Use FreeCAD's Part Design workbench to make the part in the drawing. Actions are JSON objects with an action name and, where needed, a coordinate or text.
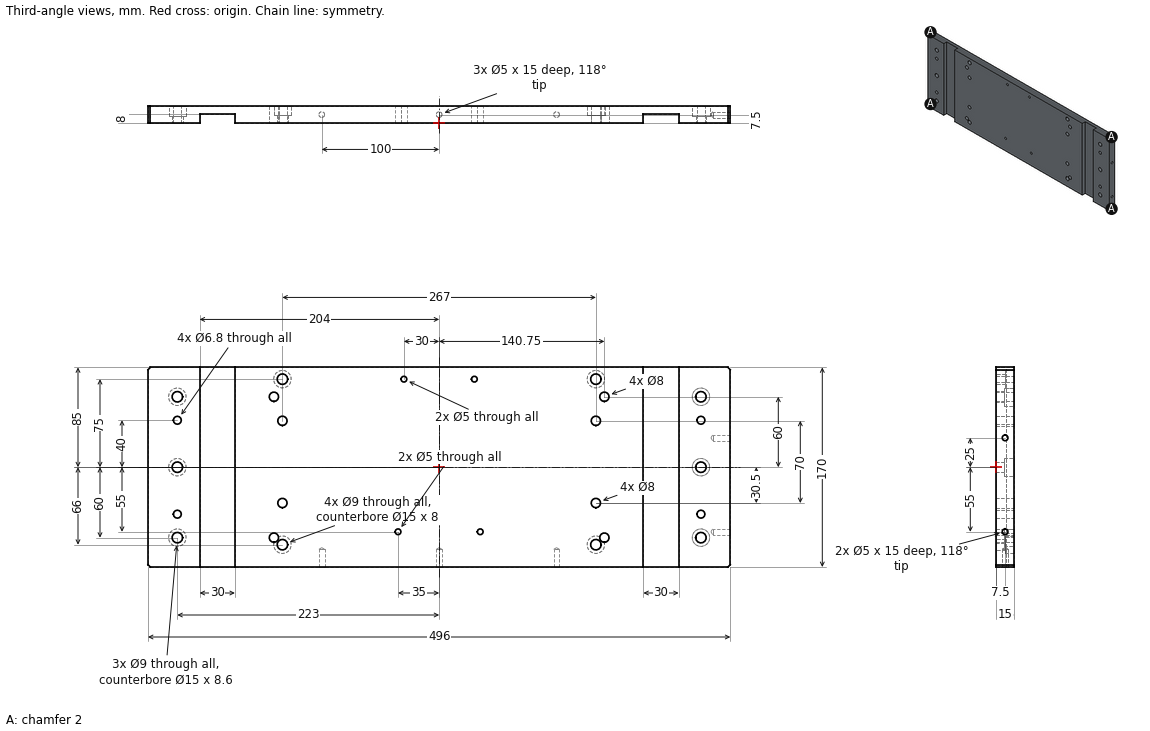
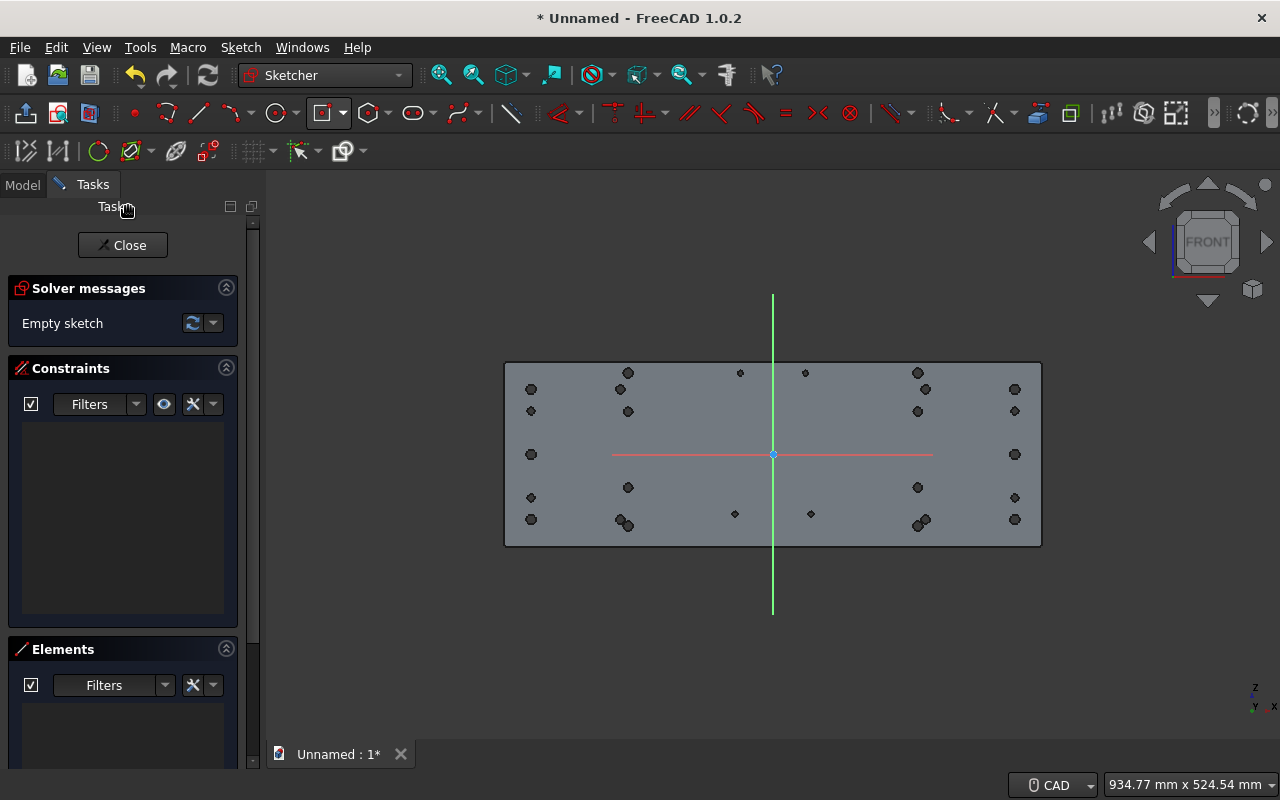
{"action": "left_click", "coordinate": [346, 114]}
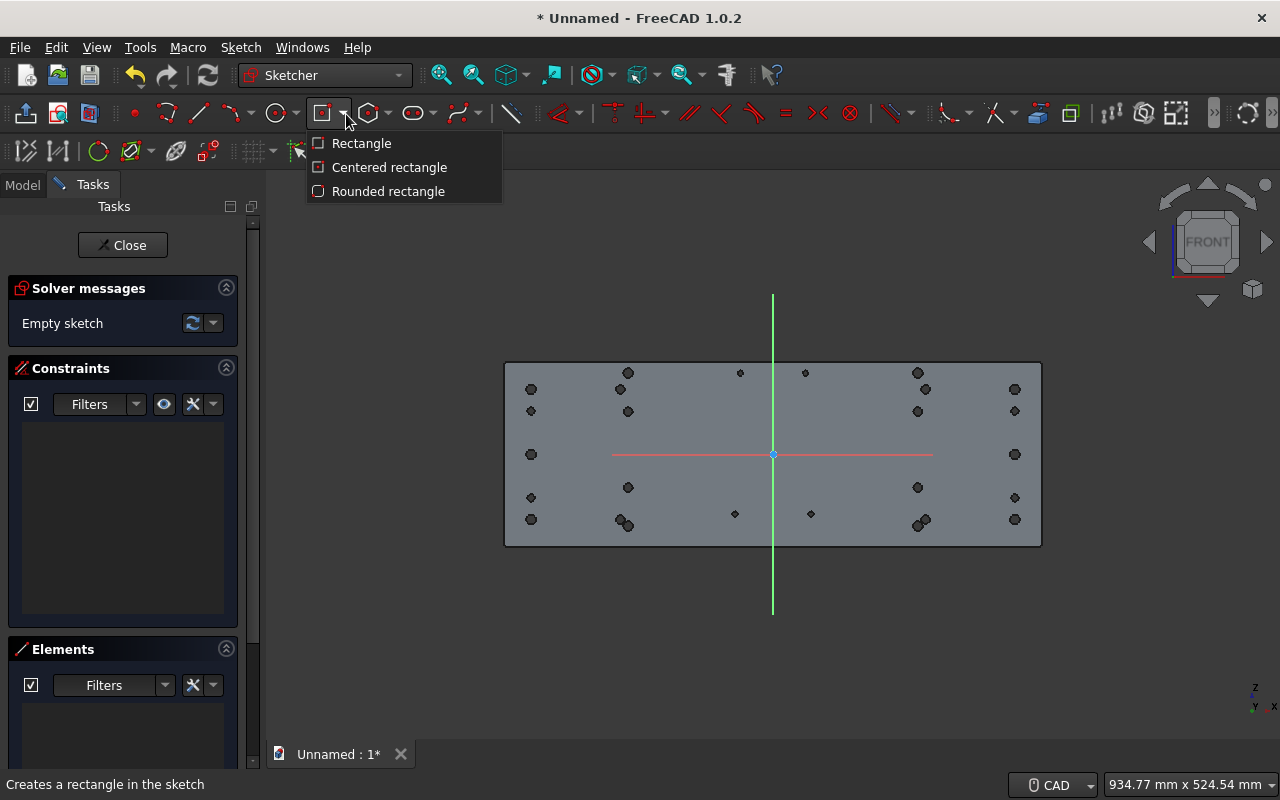
{"action": "left_click", "coordinate": [404, 143]}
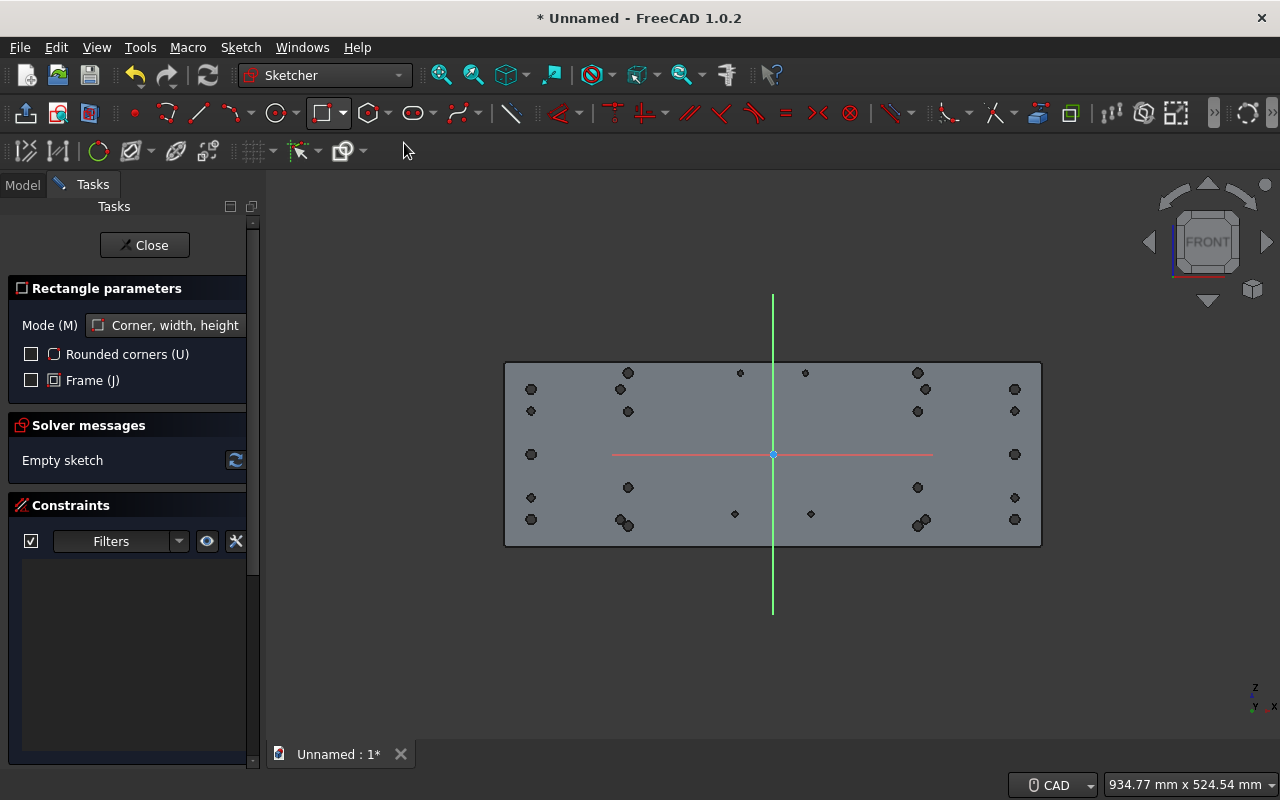
{"action": "left_click", "coordinate": [552, 362]}
{"action": "mouse_move", "coordinate": [584, 547]}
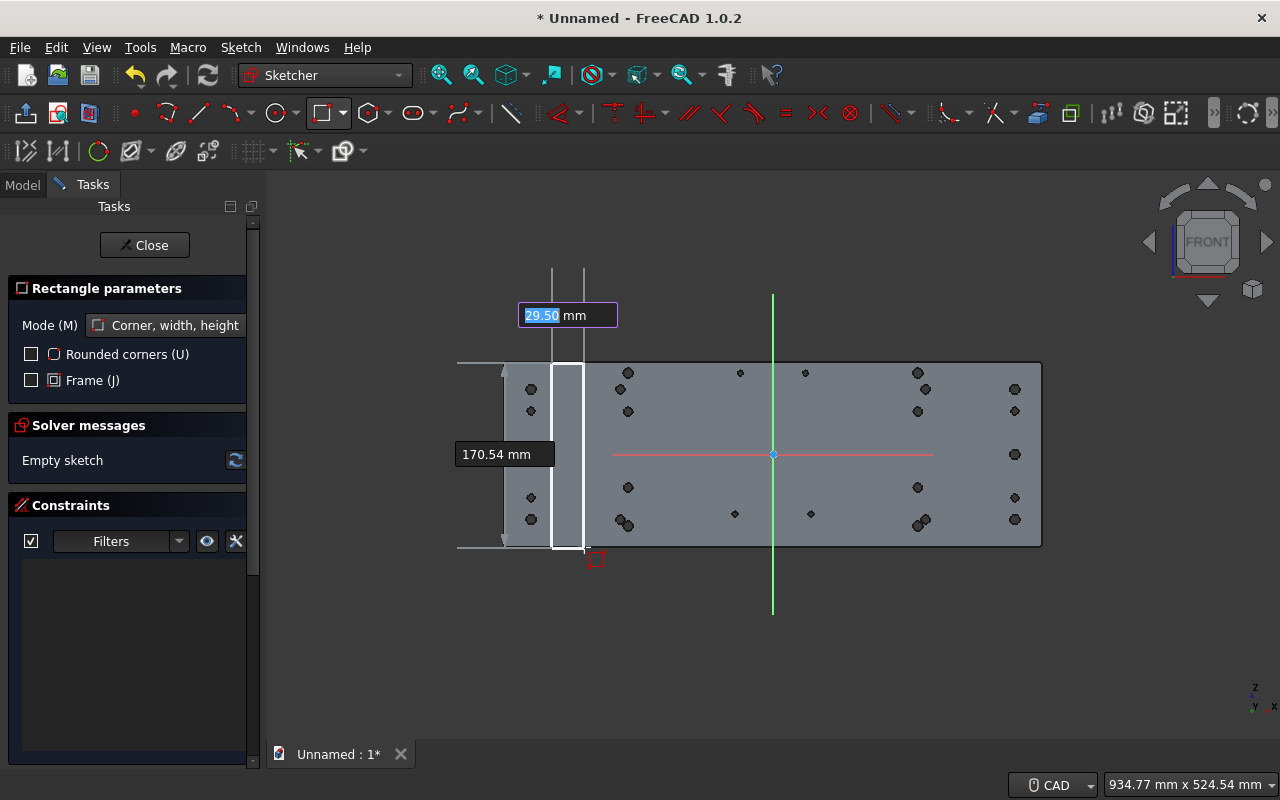
{"action": "type", "text": "30"}
{"action": "key", "text": "Tab"}
{"action": "type", "text": "170"}
{"action": "key", "text": "Return"}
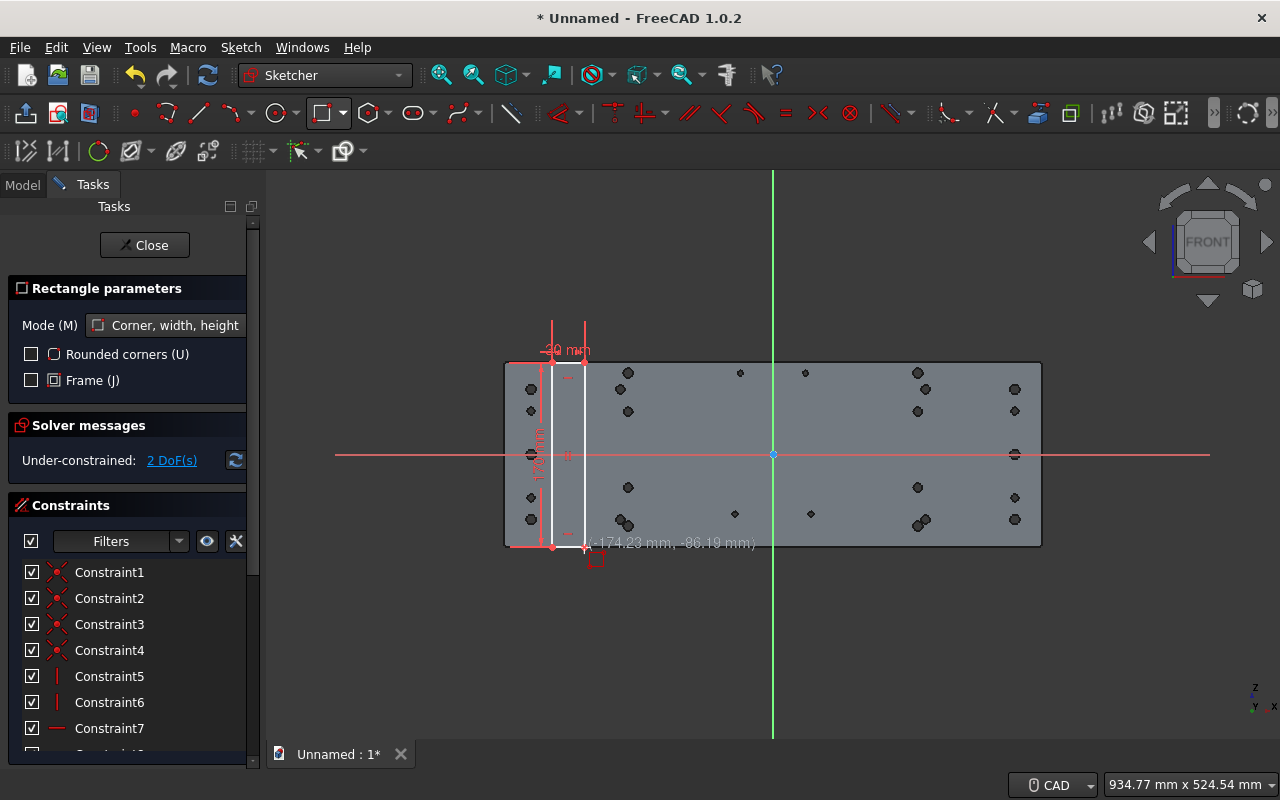
{"action": "left_click", "coordinate": [962, 362]}
{"action": "mouse_move", "coordinate": [994, 547]}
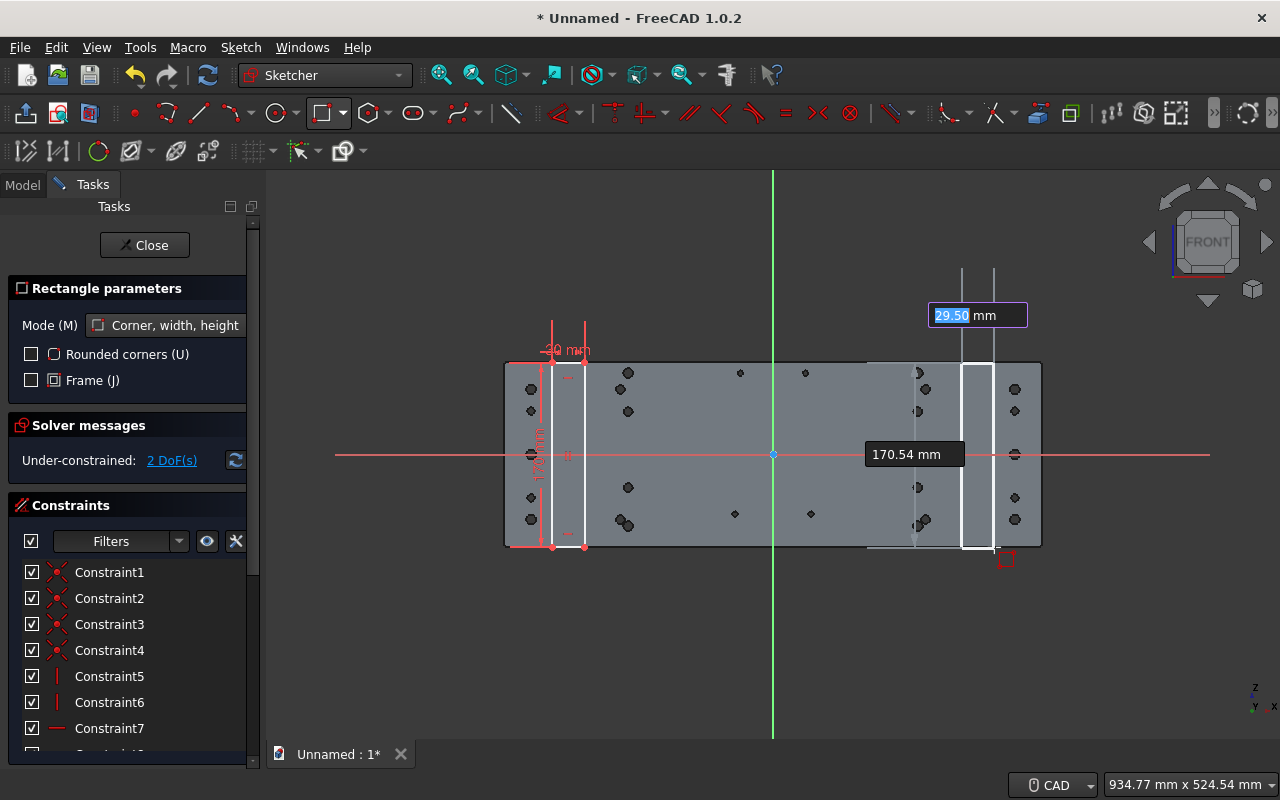
{"action": "type", "text": "30"}
{"action": "key", "text": "Tab"}
{"action": "type", "text": "170"}
{"action": "key", "text": "Return"}
{"action": "key", "text": "Escape"}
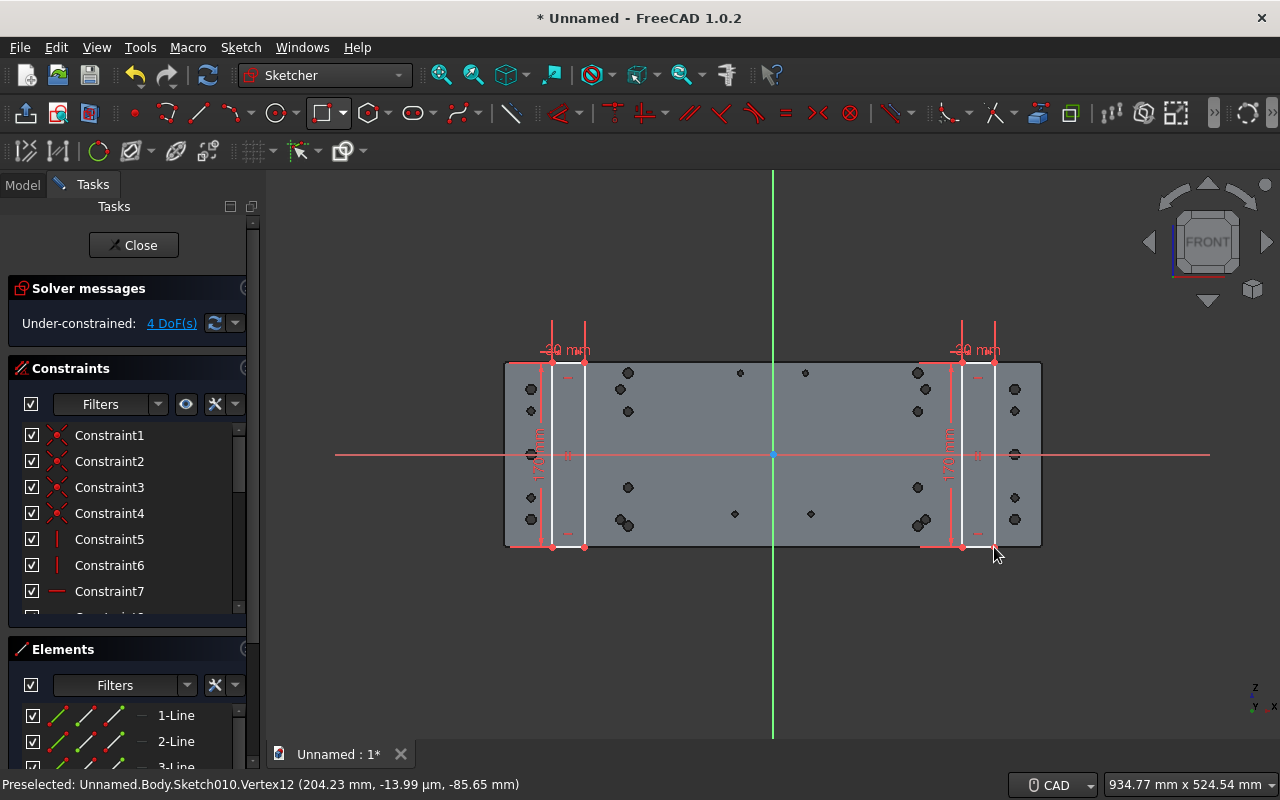
{"action": "left_click", "coordinate": [585, 363]}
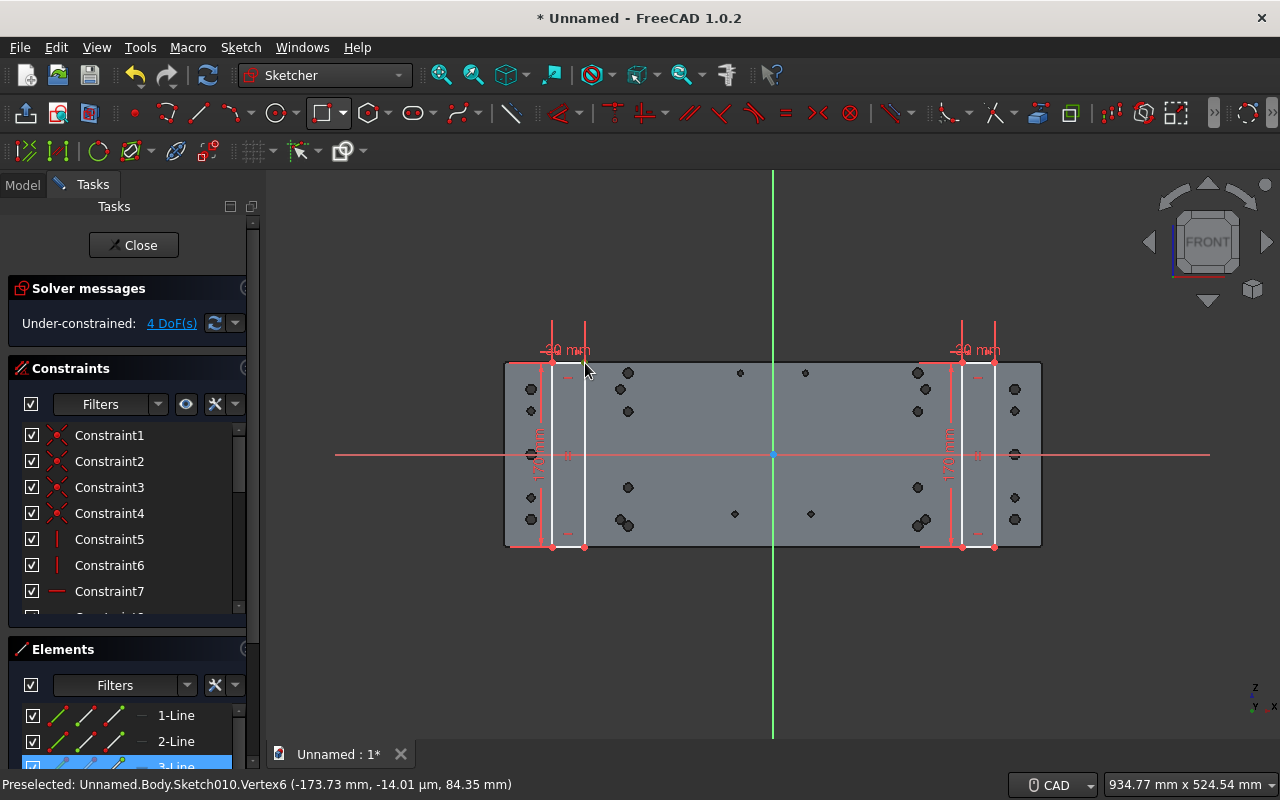
{"action": "left_click", "coordinate": [962, 363]}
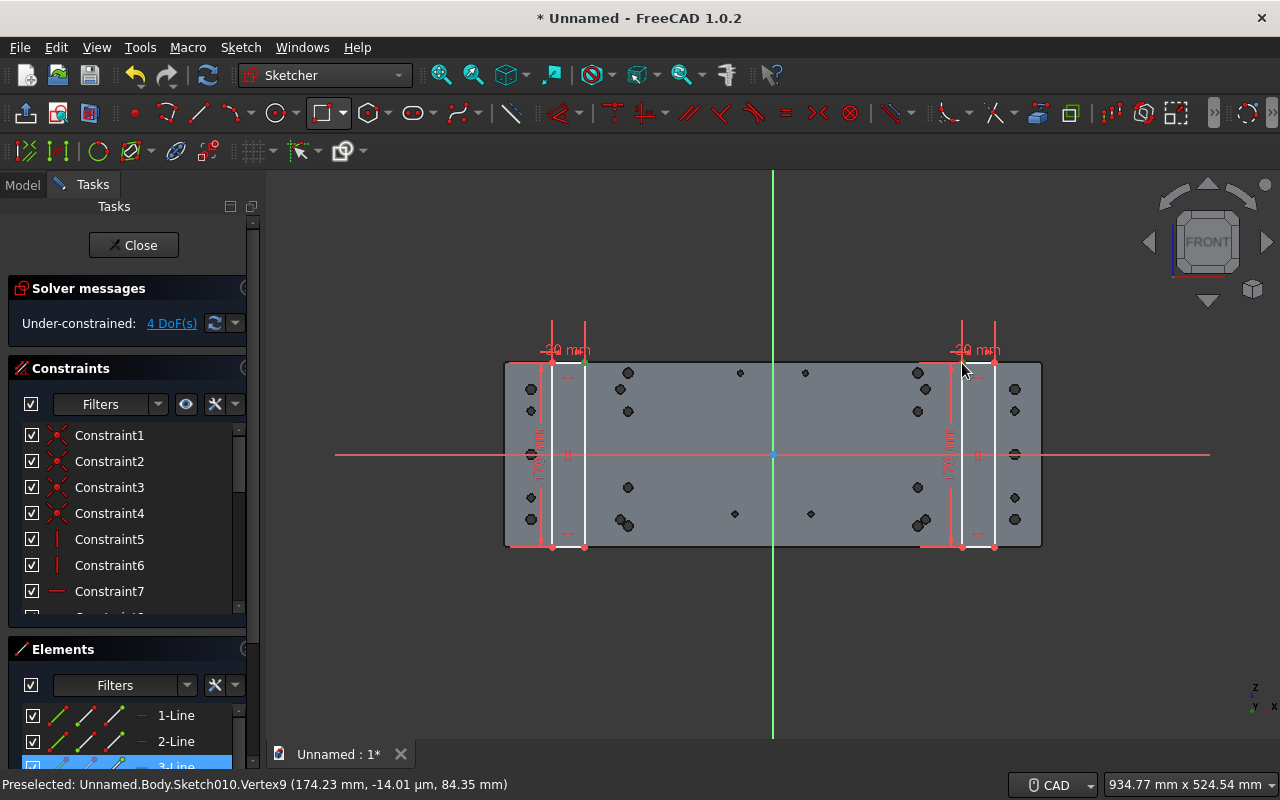
{"action": "left_click", "coordinate": [773, 674]}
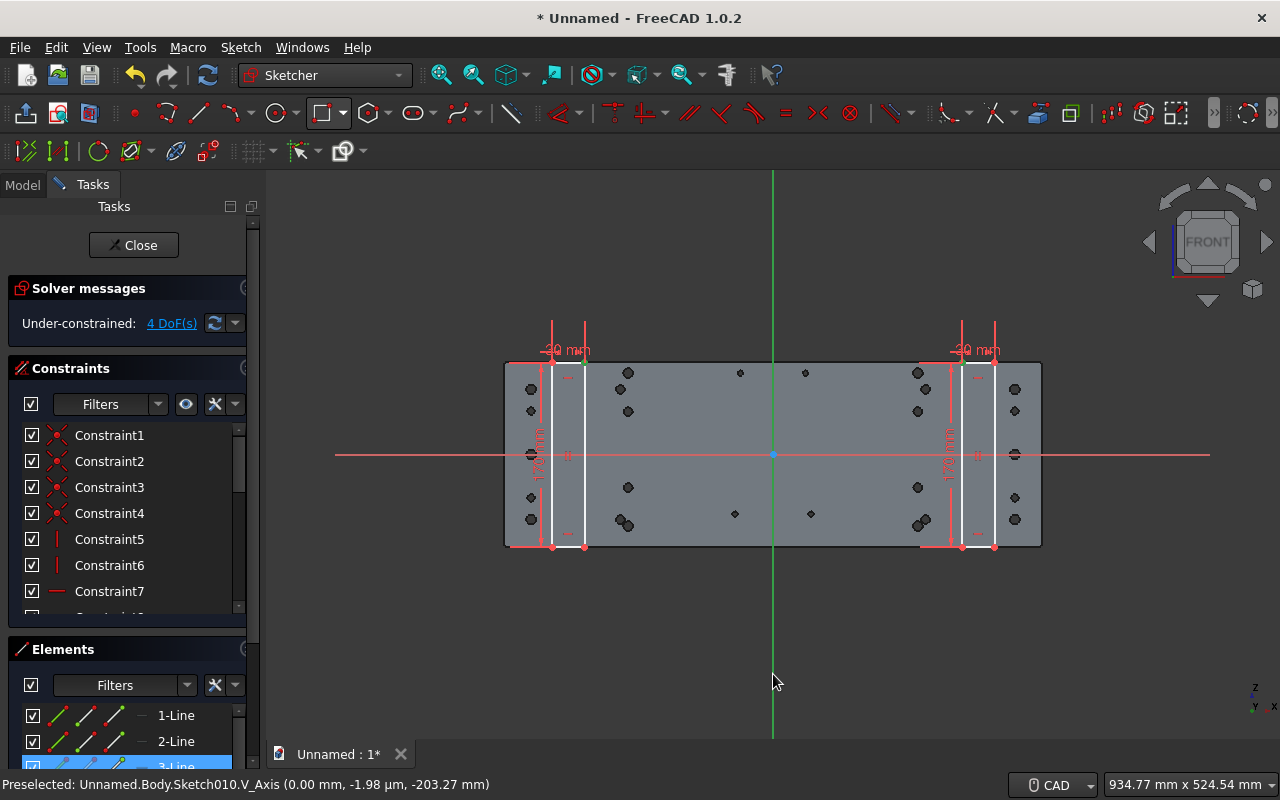
{"action": "left_click", "coordinate": [818, 114]}